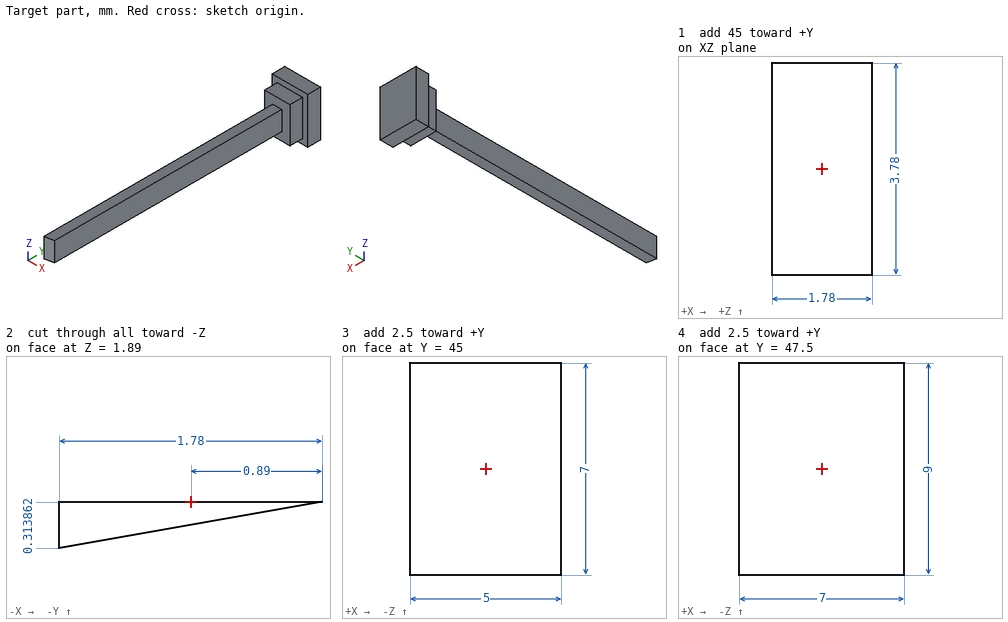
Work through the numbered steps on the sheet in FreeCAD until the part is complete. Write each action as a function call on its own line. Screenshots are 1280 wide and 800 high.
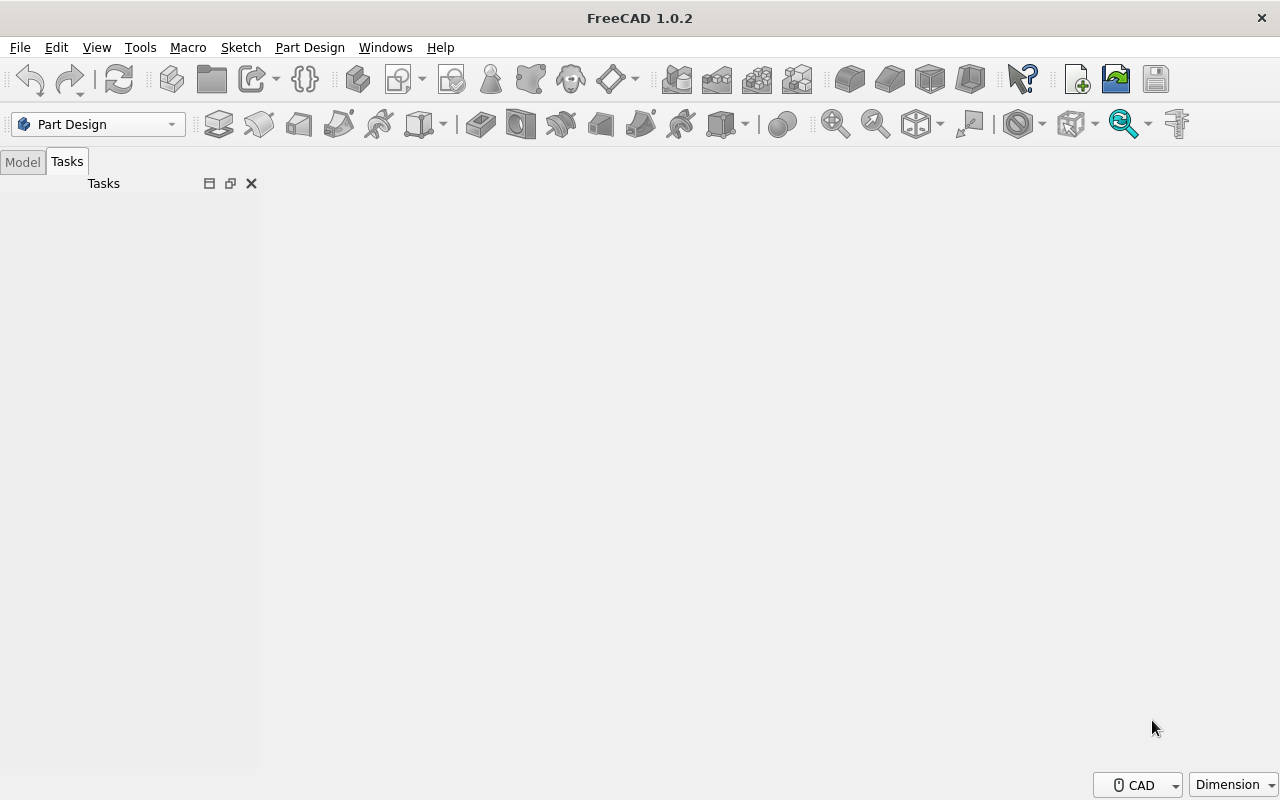
key(ctrl+n)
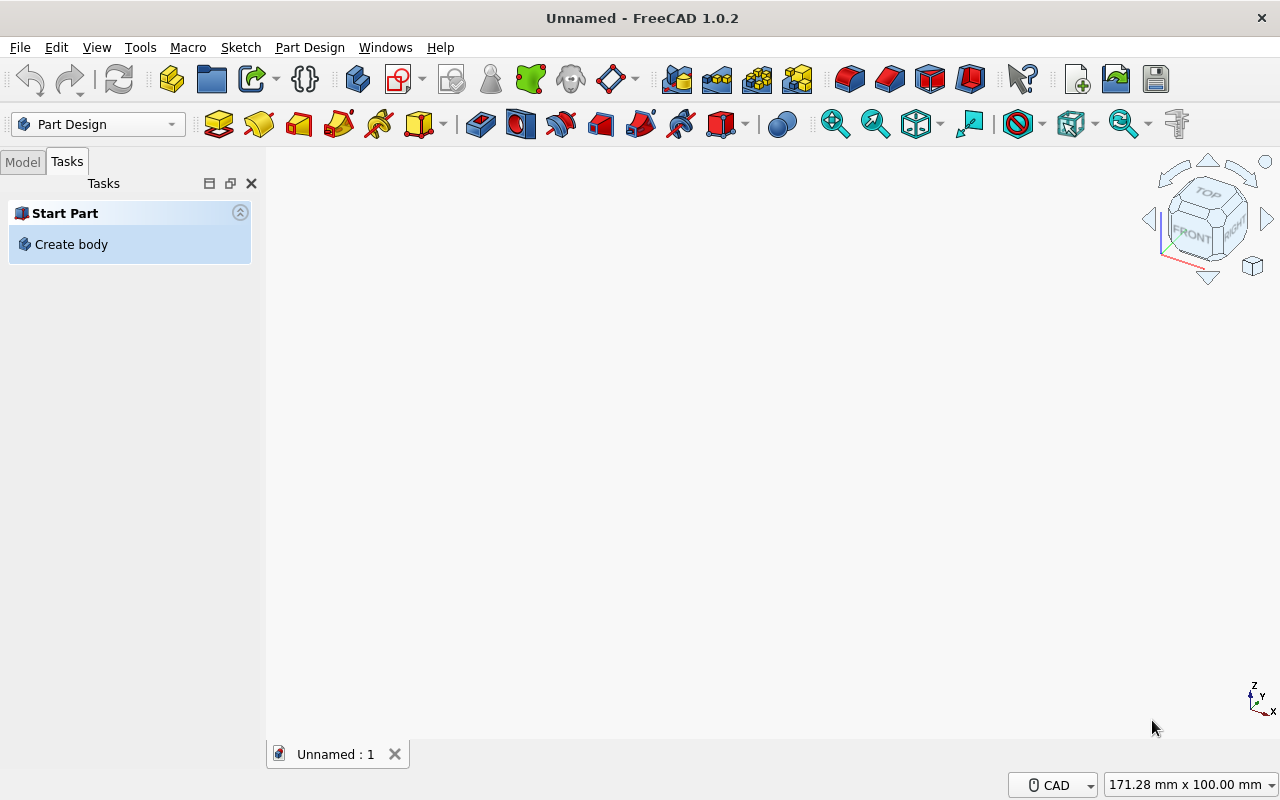
click(398, 80)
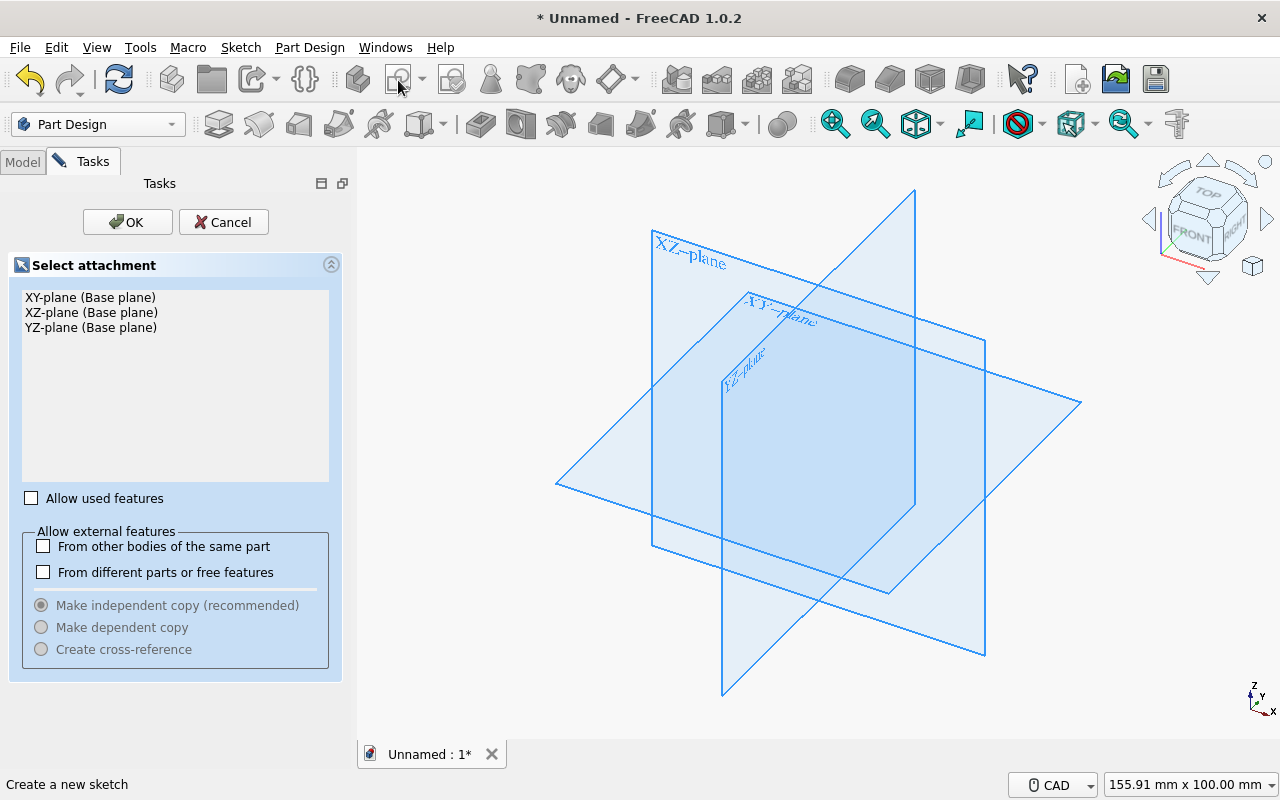
click(82, 312)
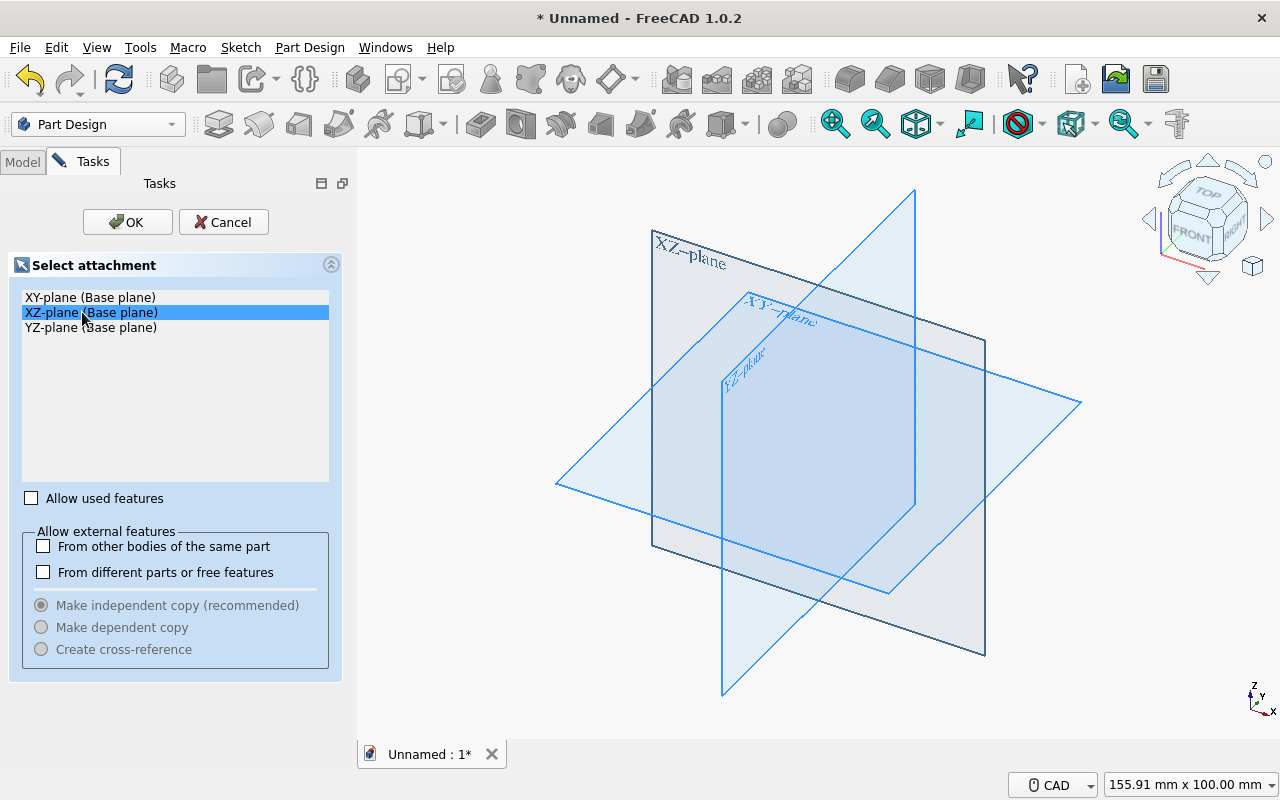
click(128, 222)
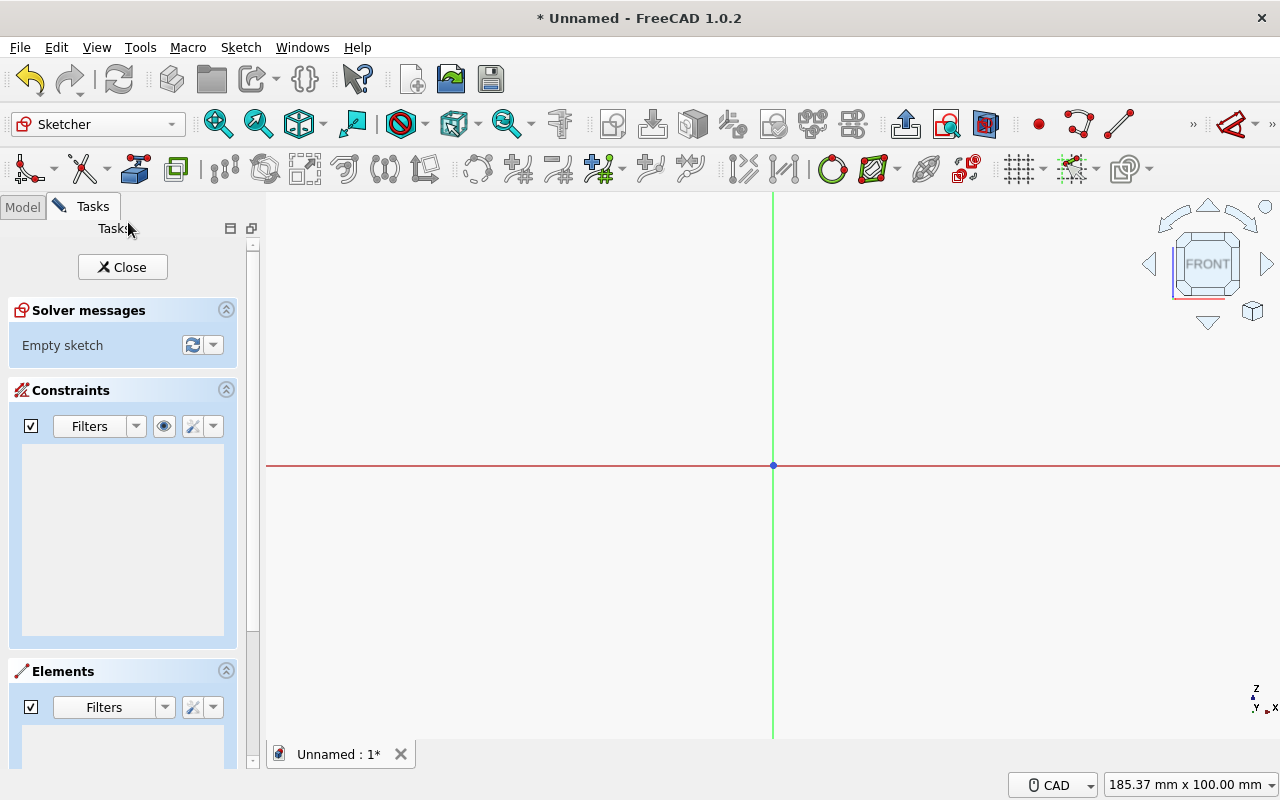
scroll(777, 466, up, 14)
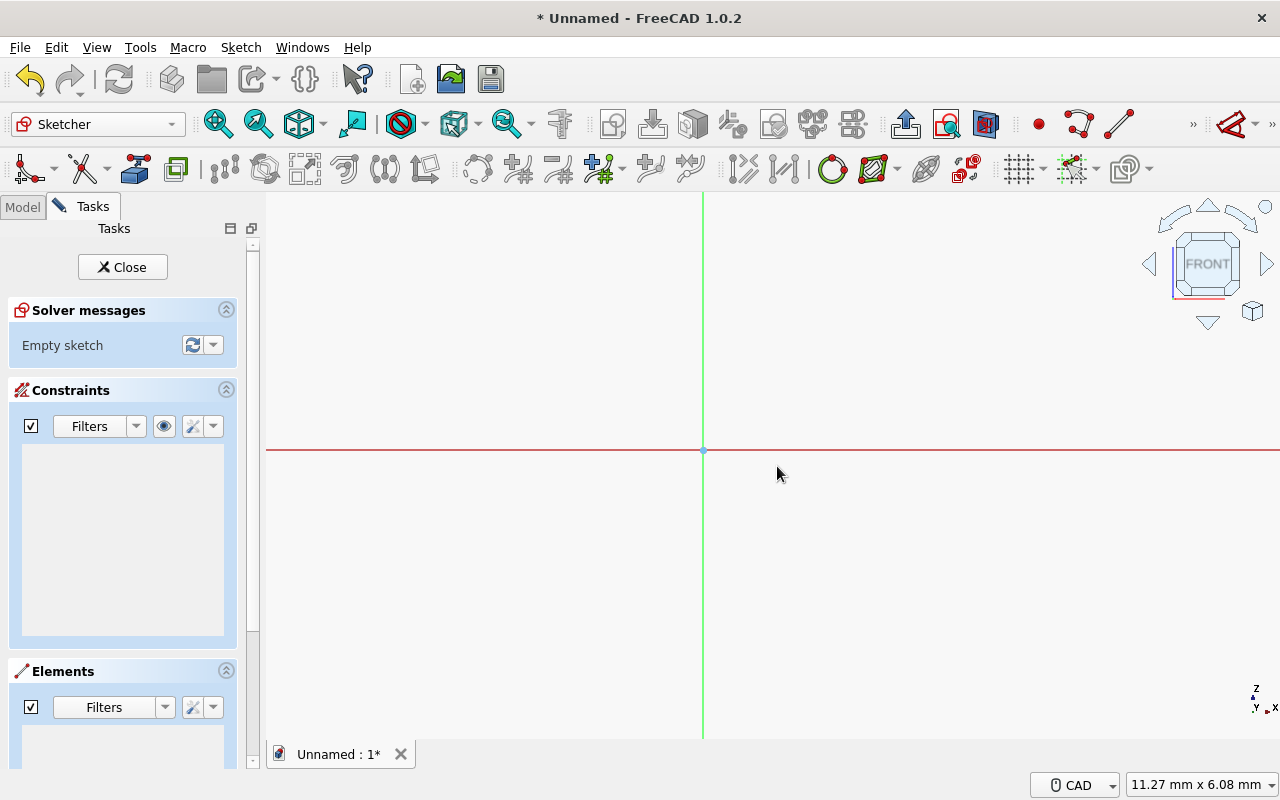
key(g)
key(v)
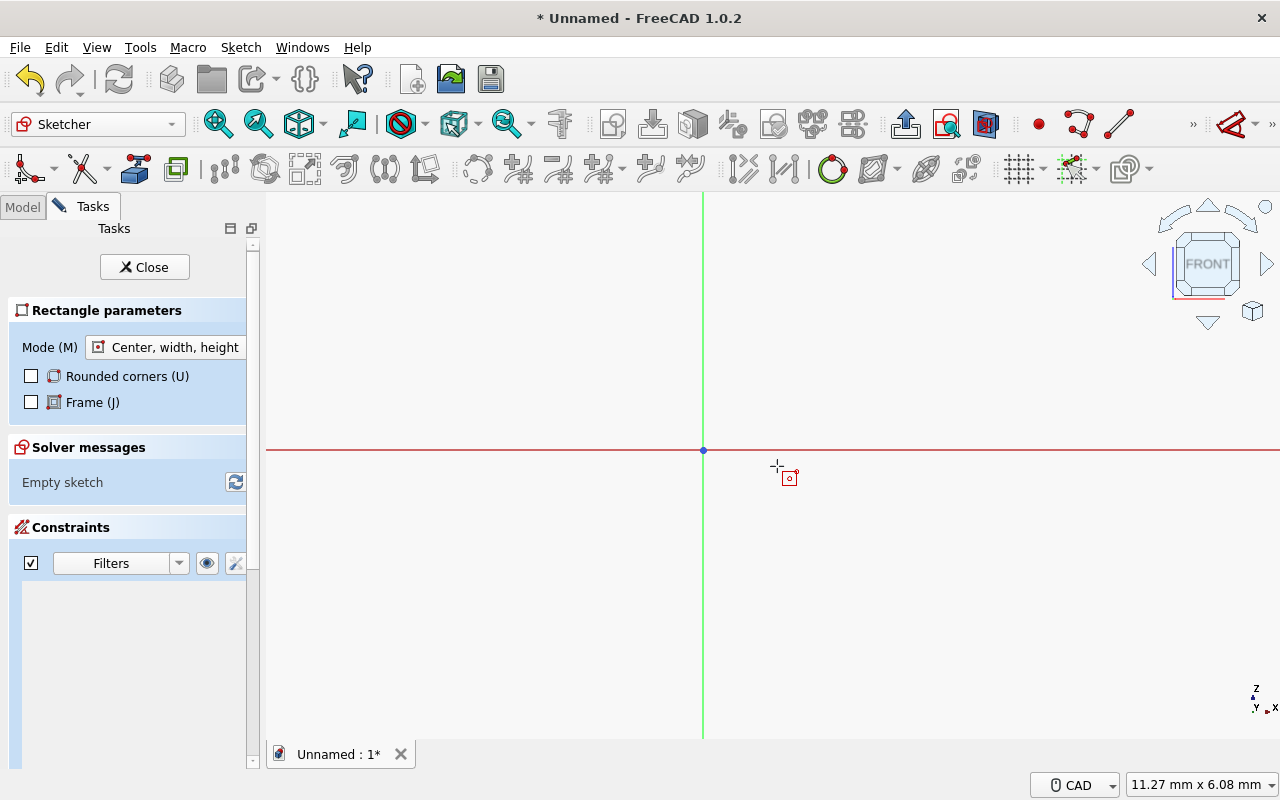
click(703, 450)
click(783, 280)
key(Escape)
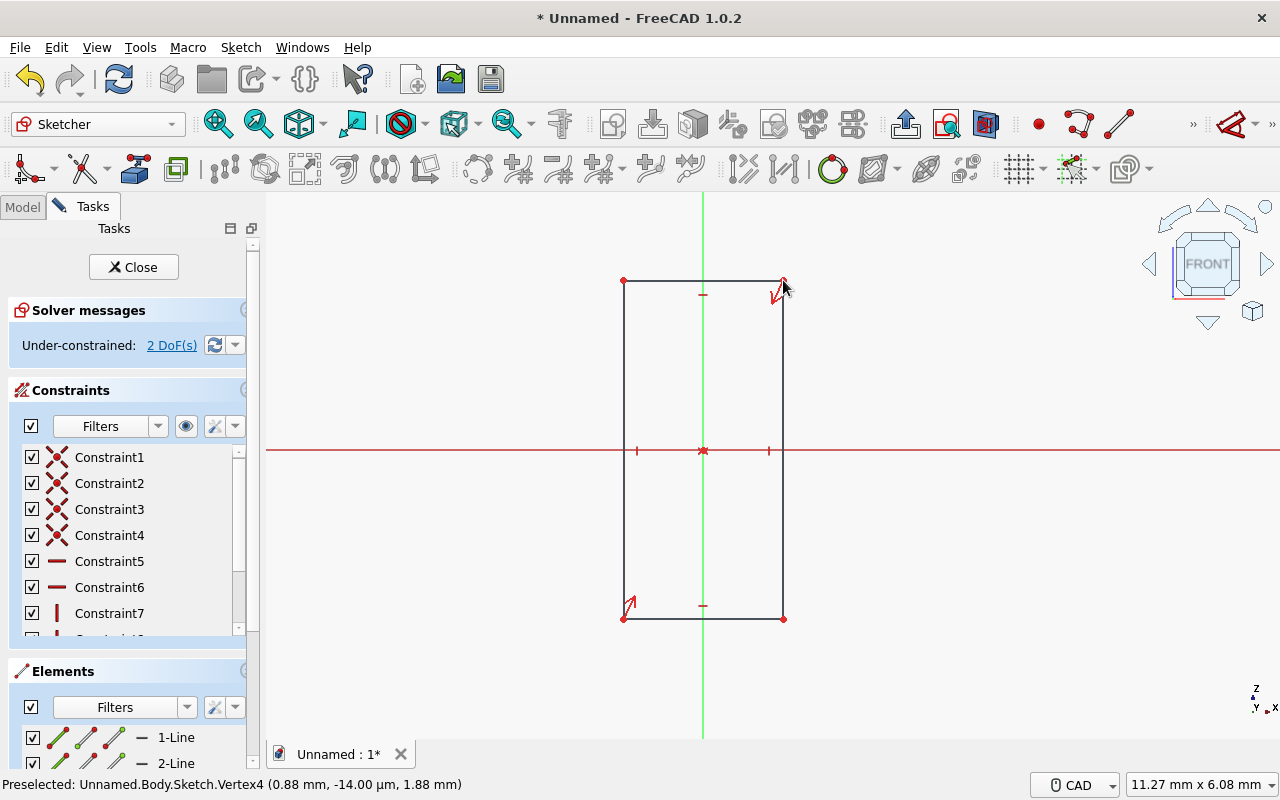
key(d)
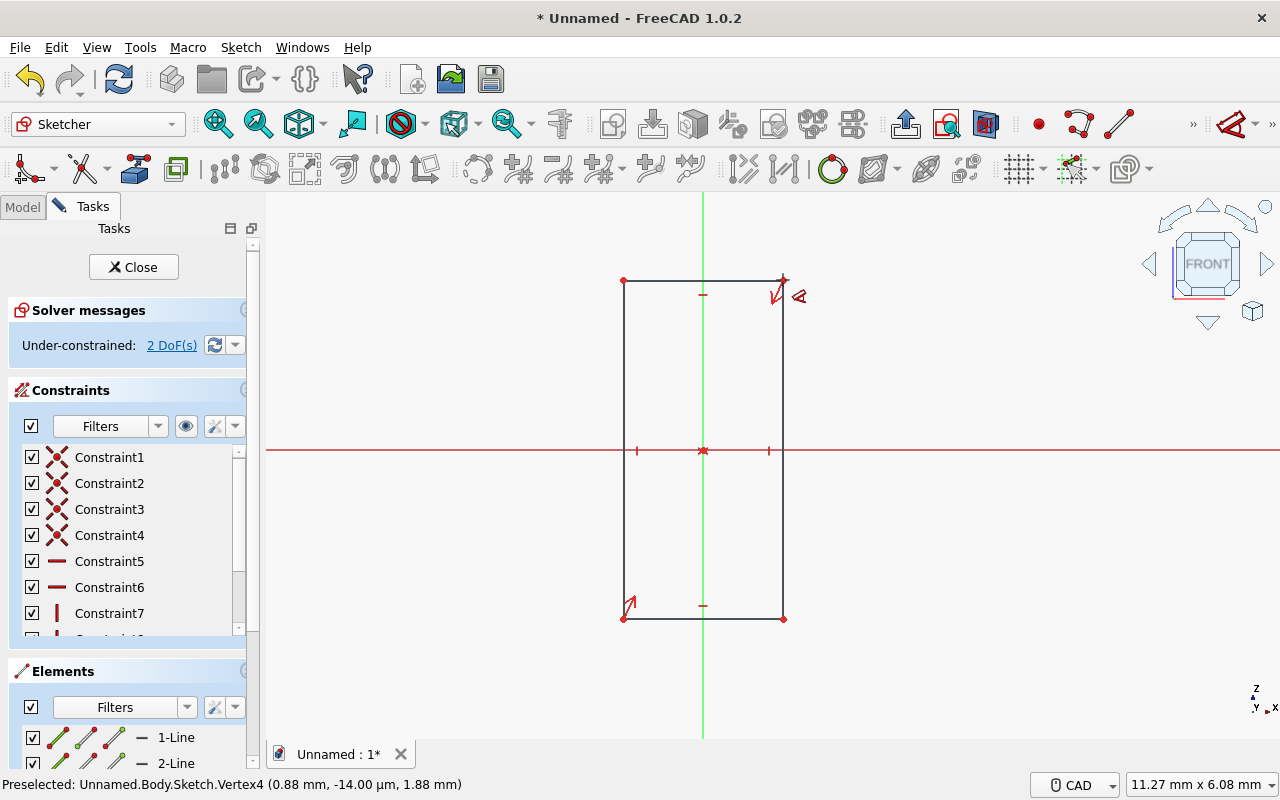
click(672, 619)
click(667, 653)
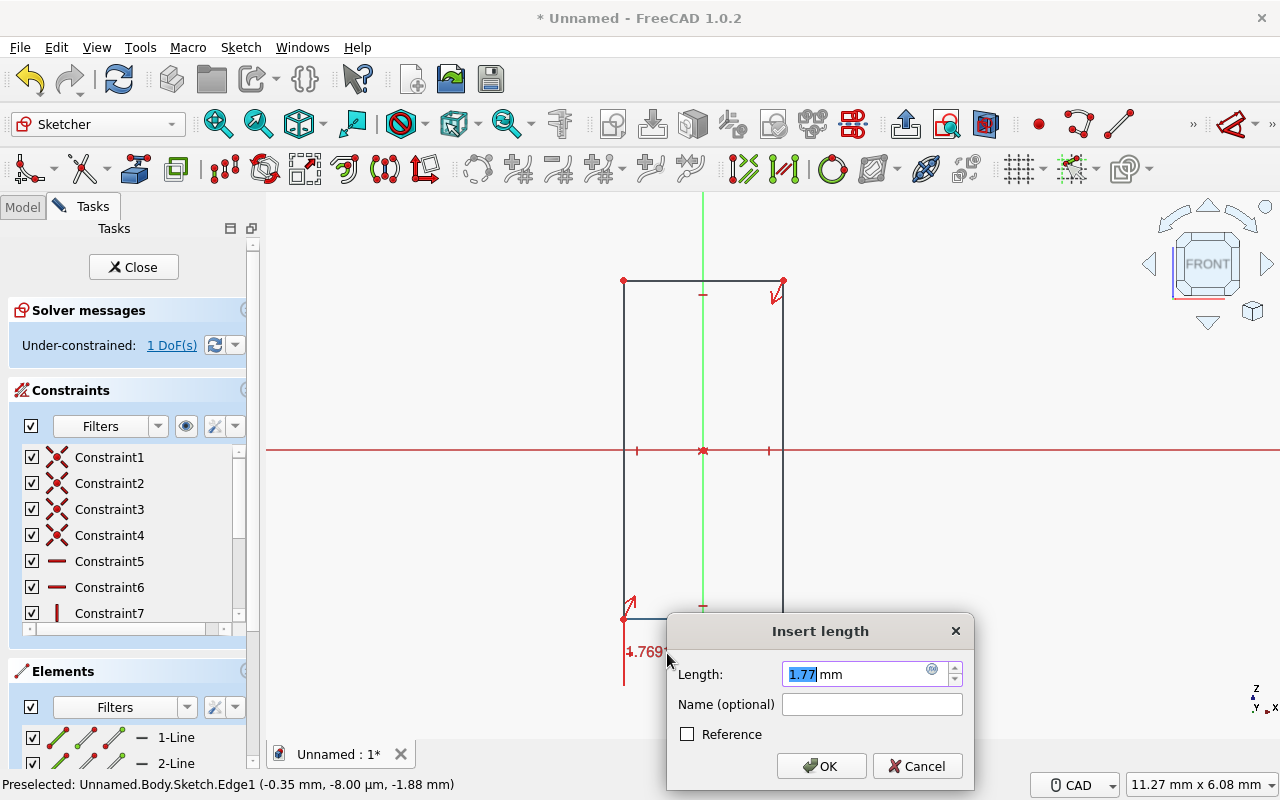
text(1.78)
key(Return)